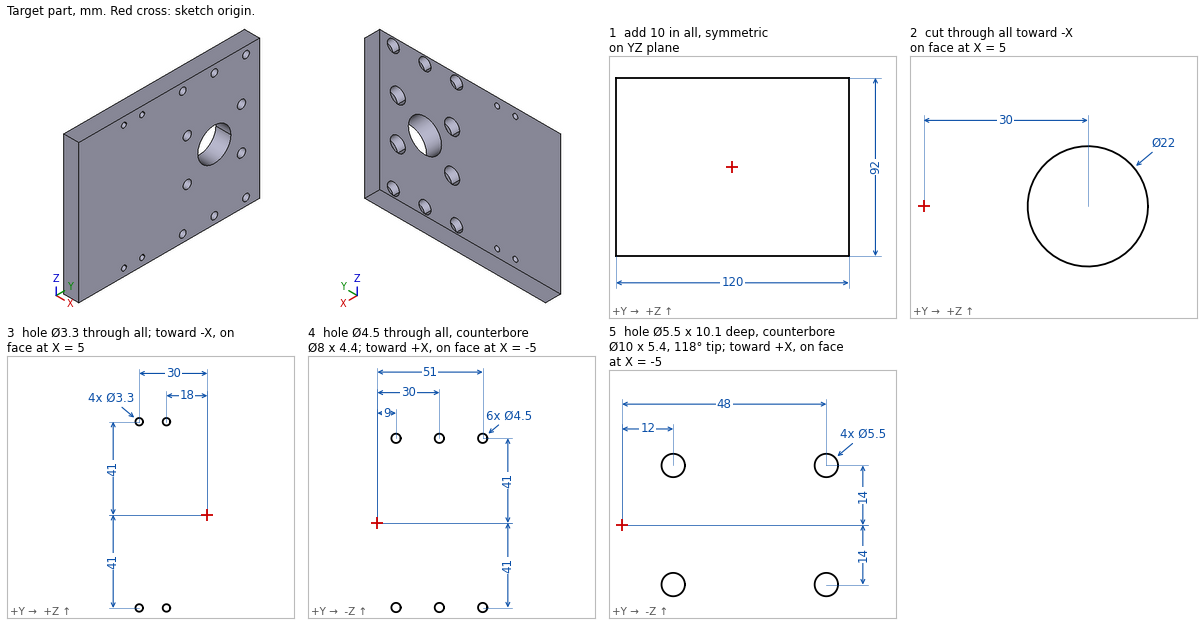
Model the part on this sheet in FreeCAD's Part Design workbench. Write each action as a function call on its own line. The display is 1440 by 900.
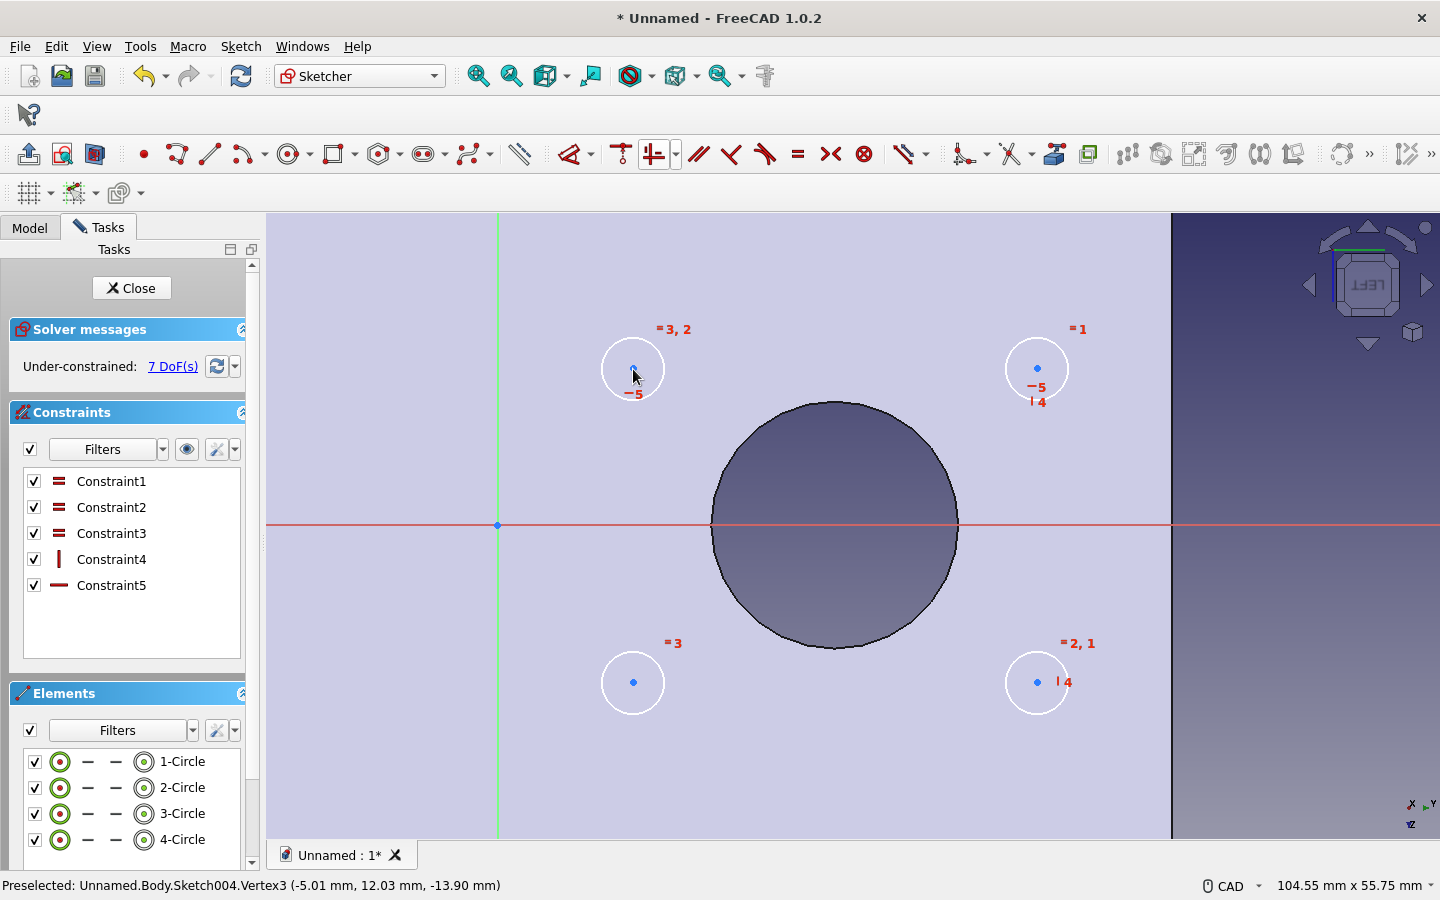
click(633, 369)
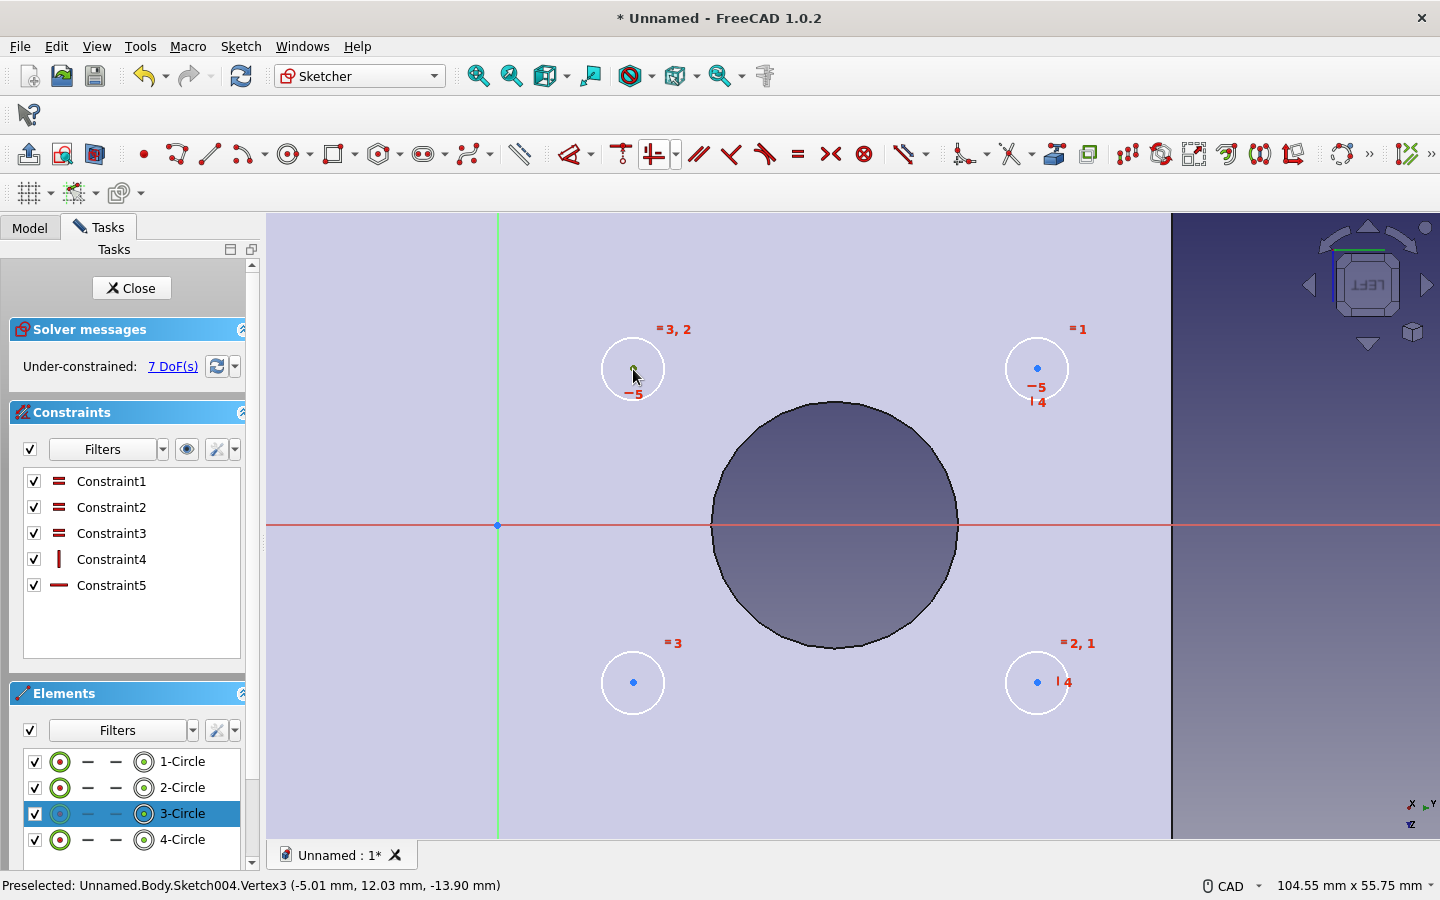
click(633, 683)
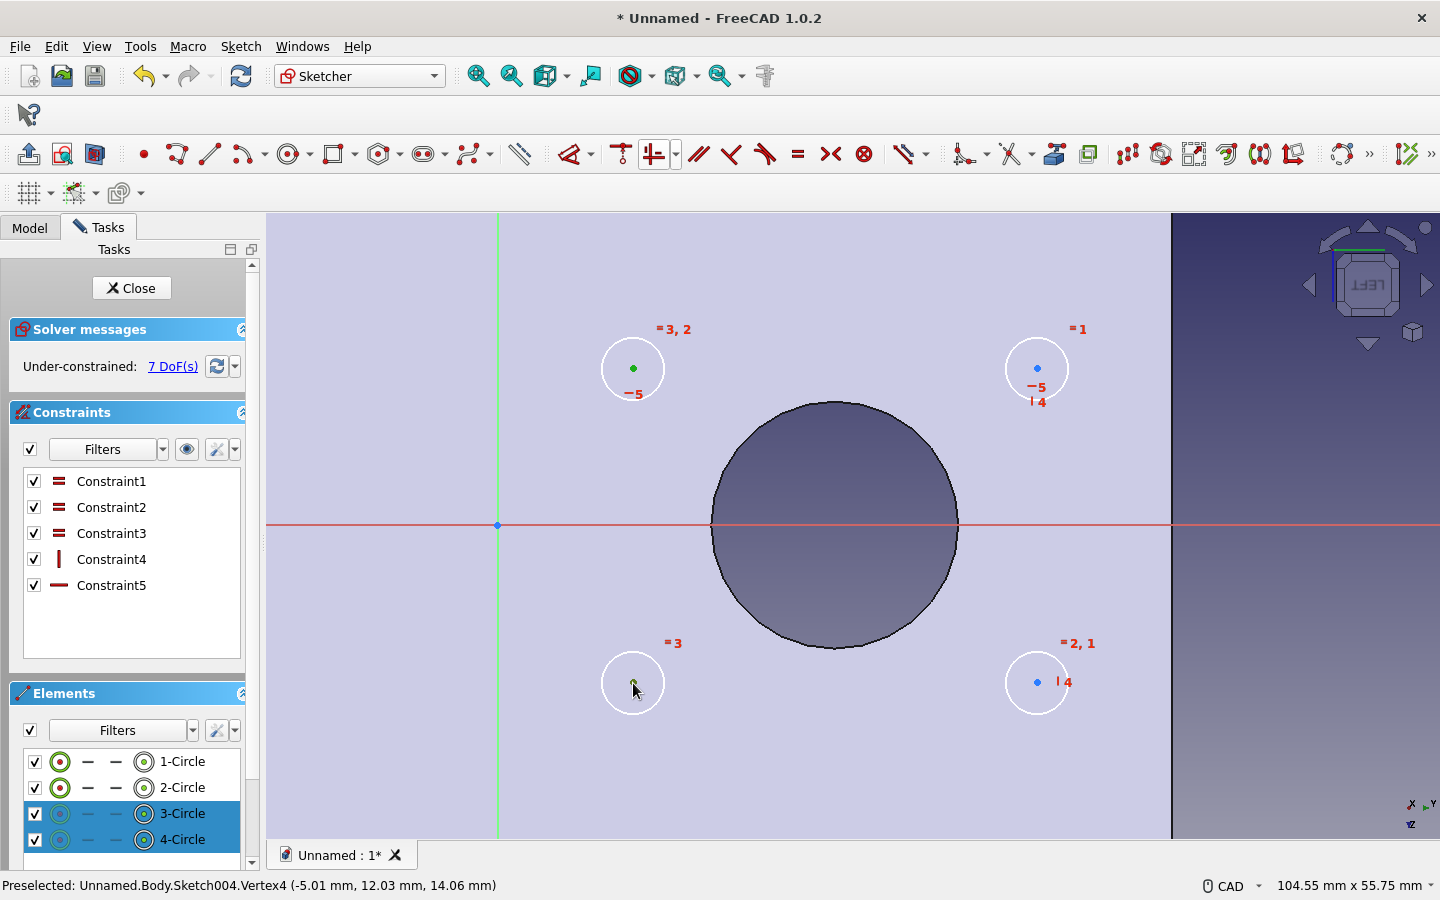
key(v)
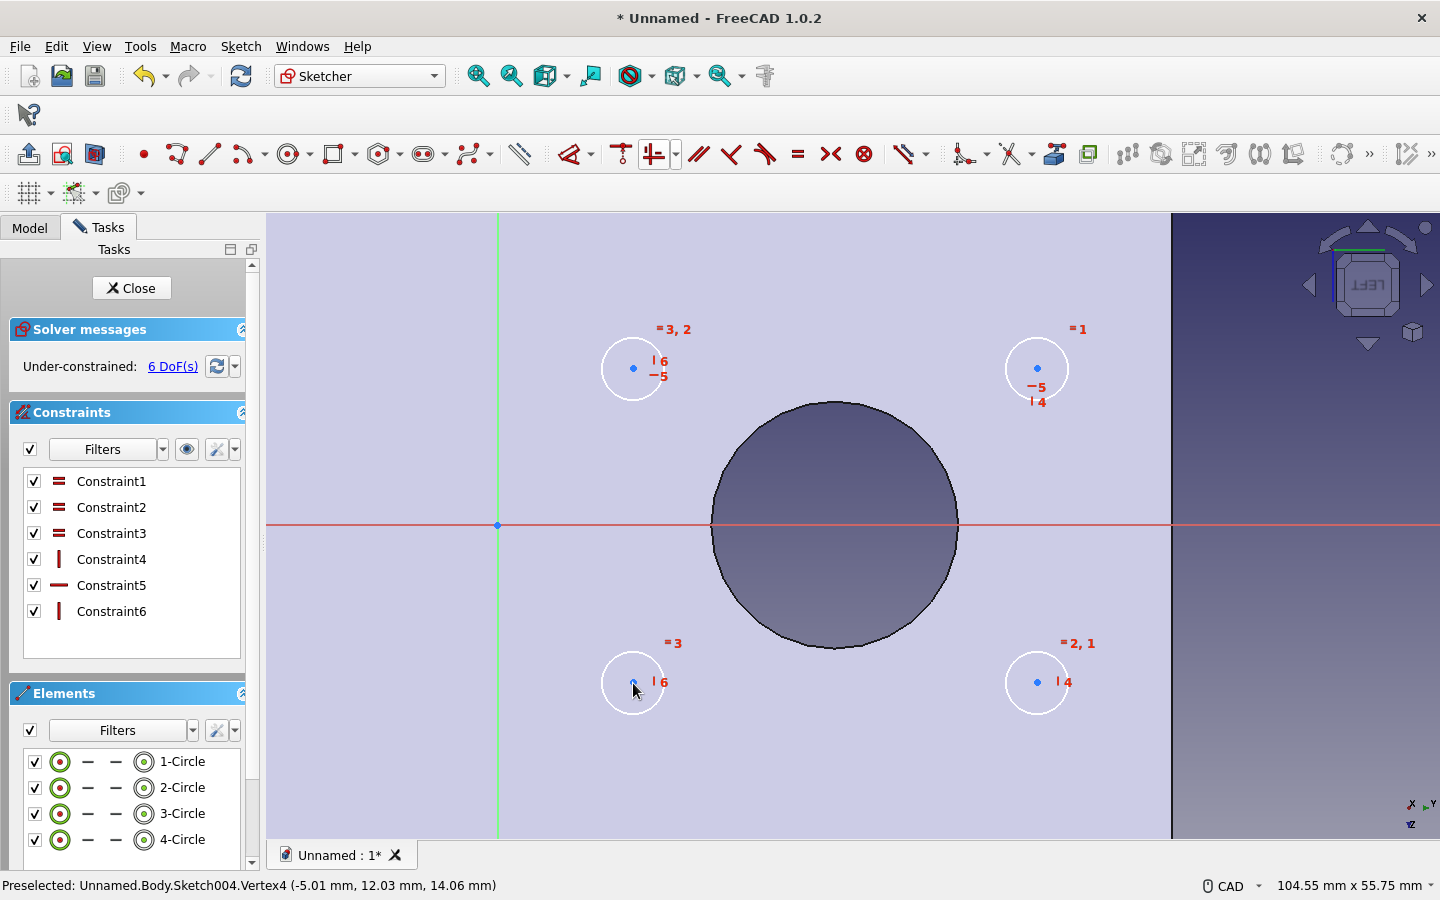
click(1037, 683)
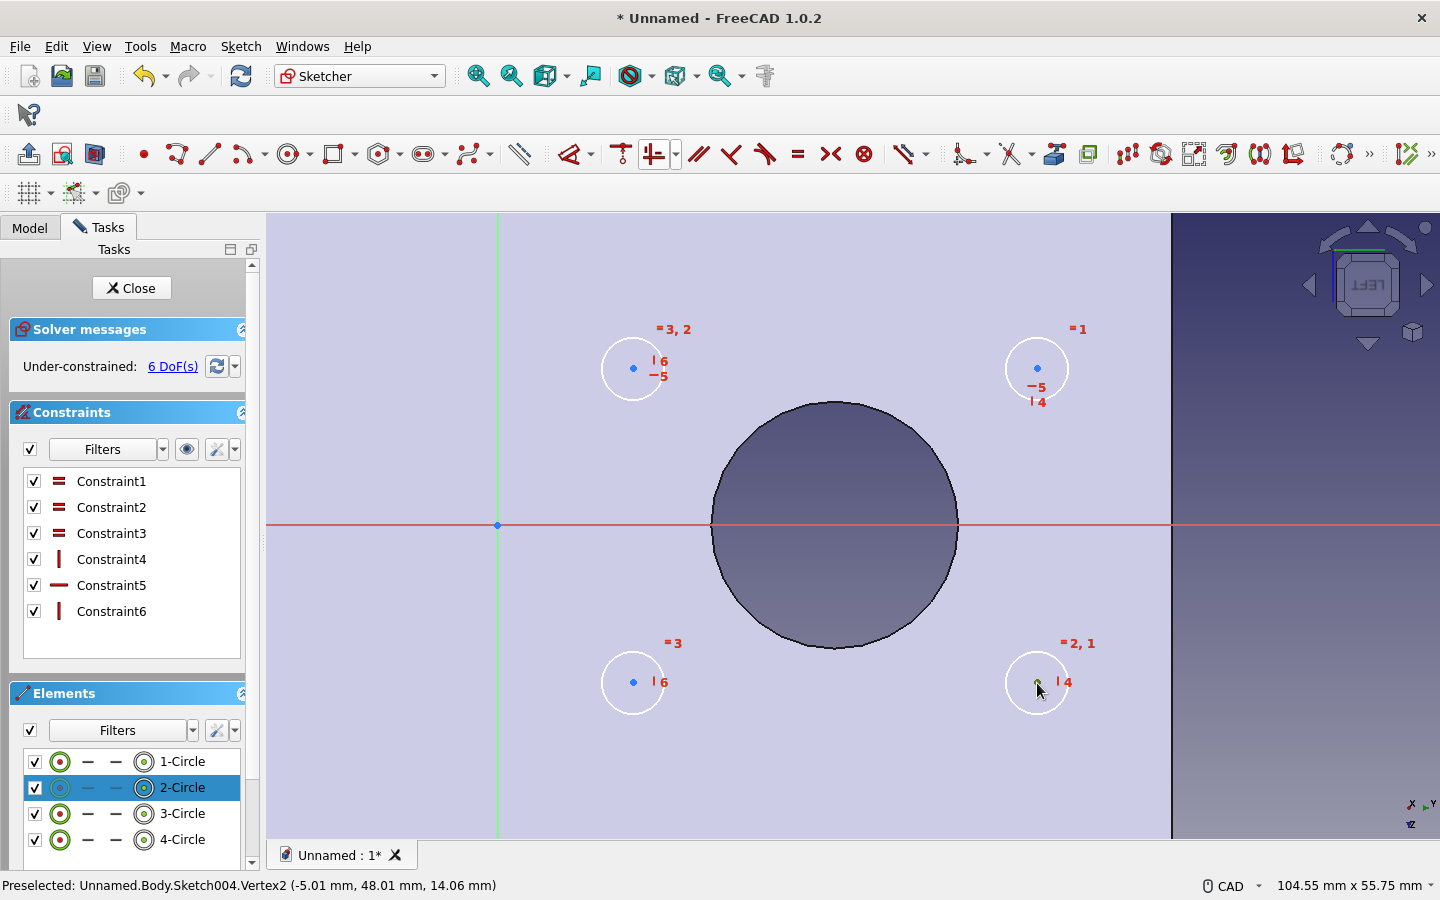
click(633, 683)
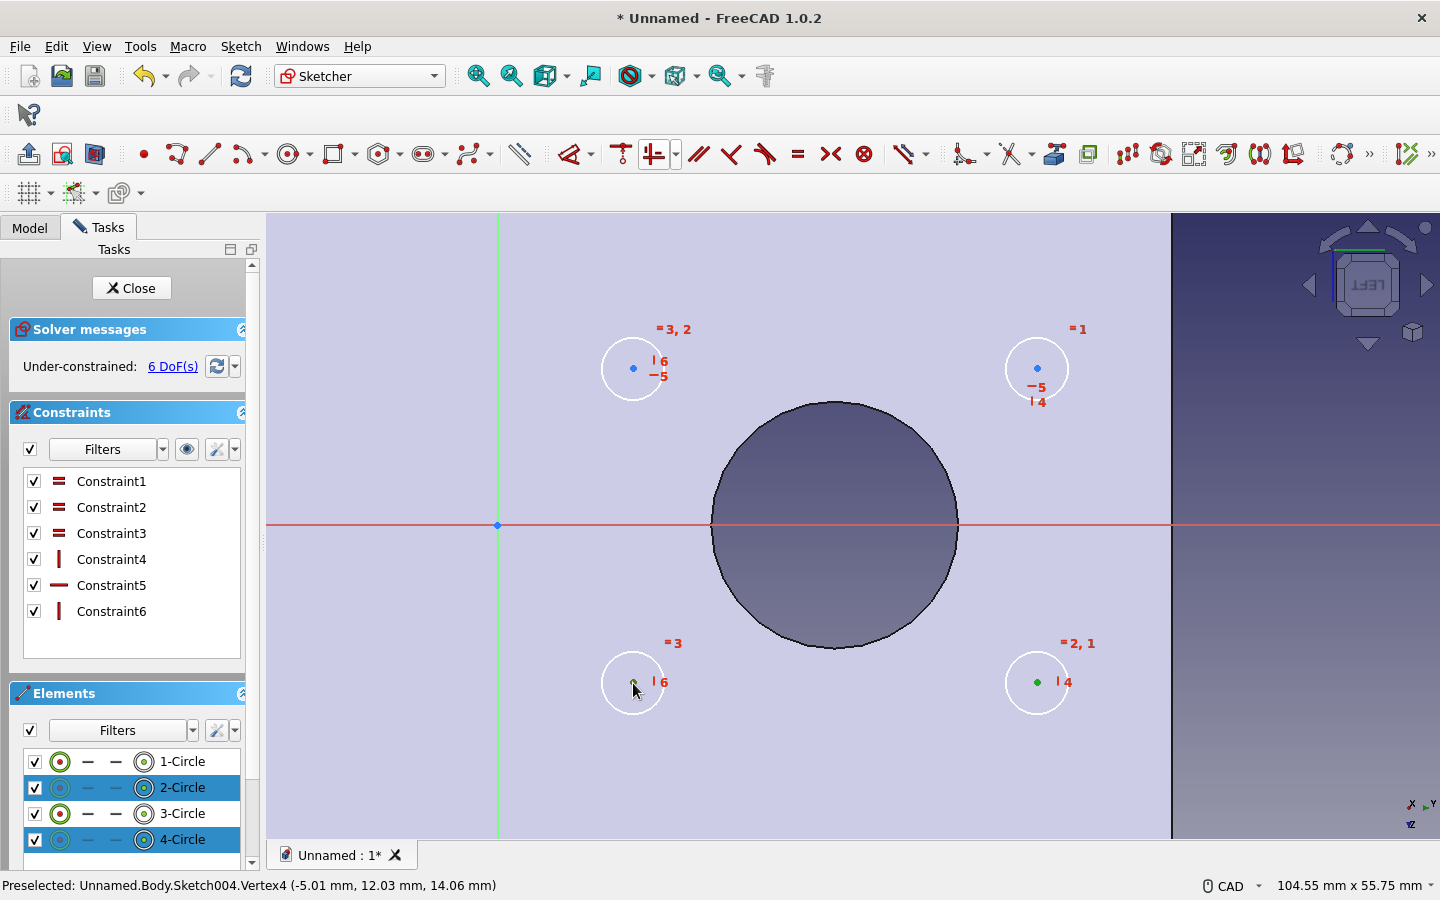
click(676, 154)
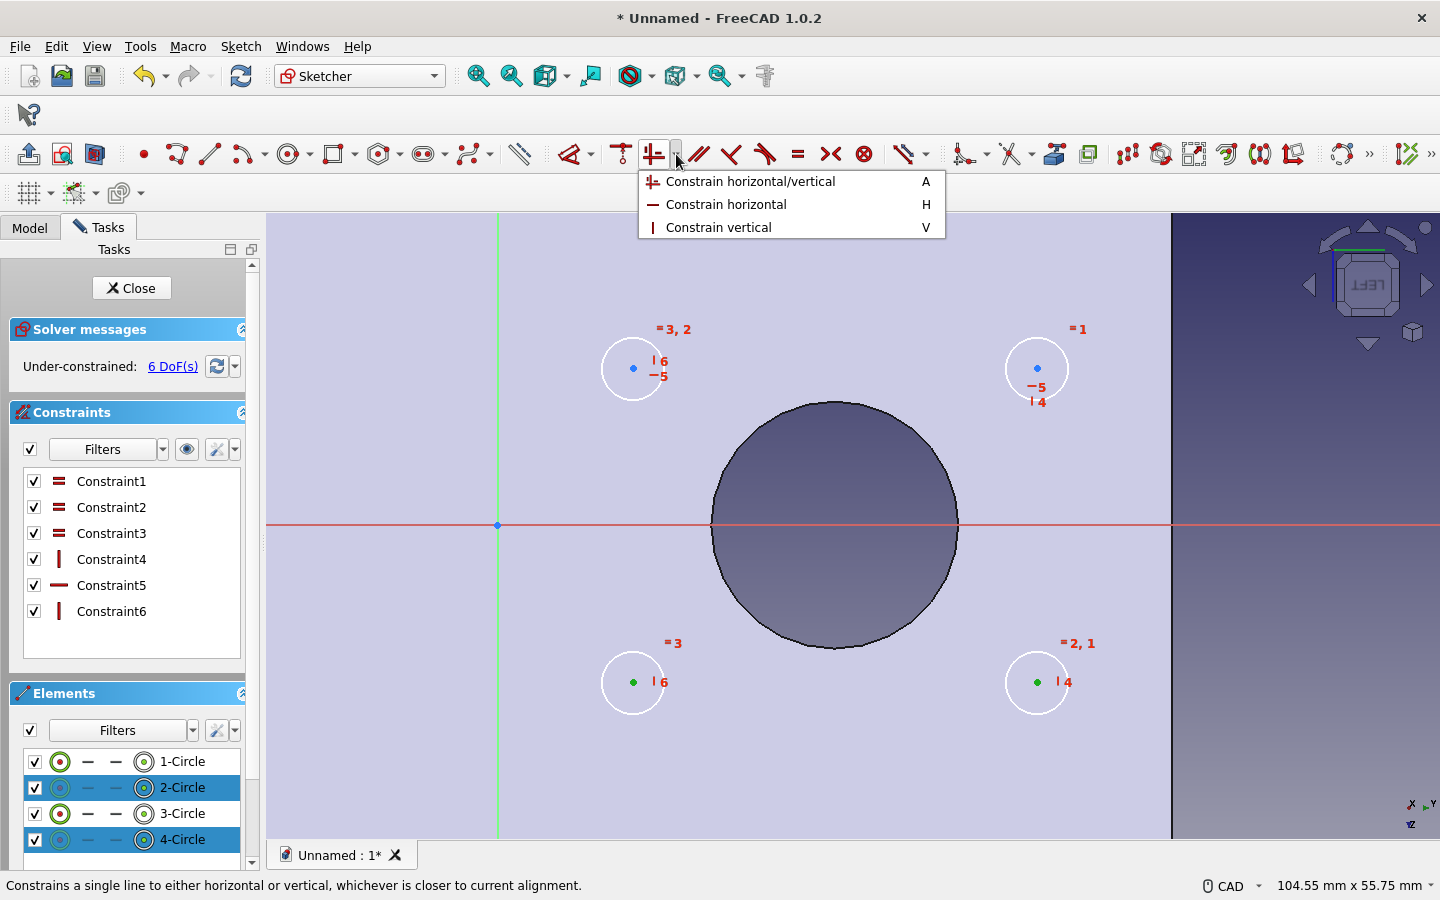
click(792, 204)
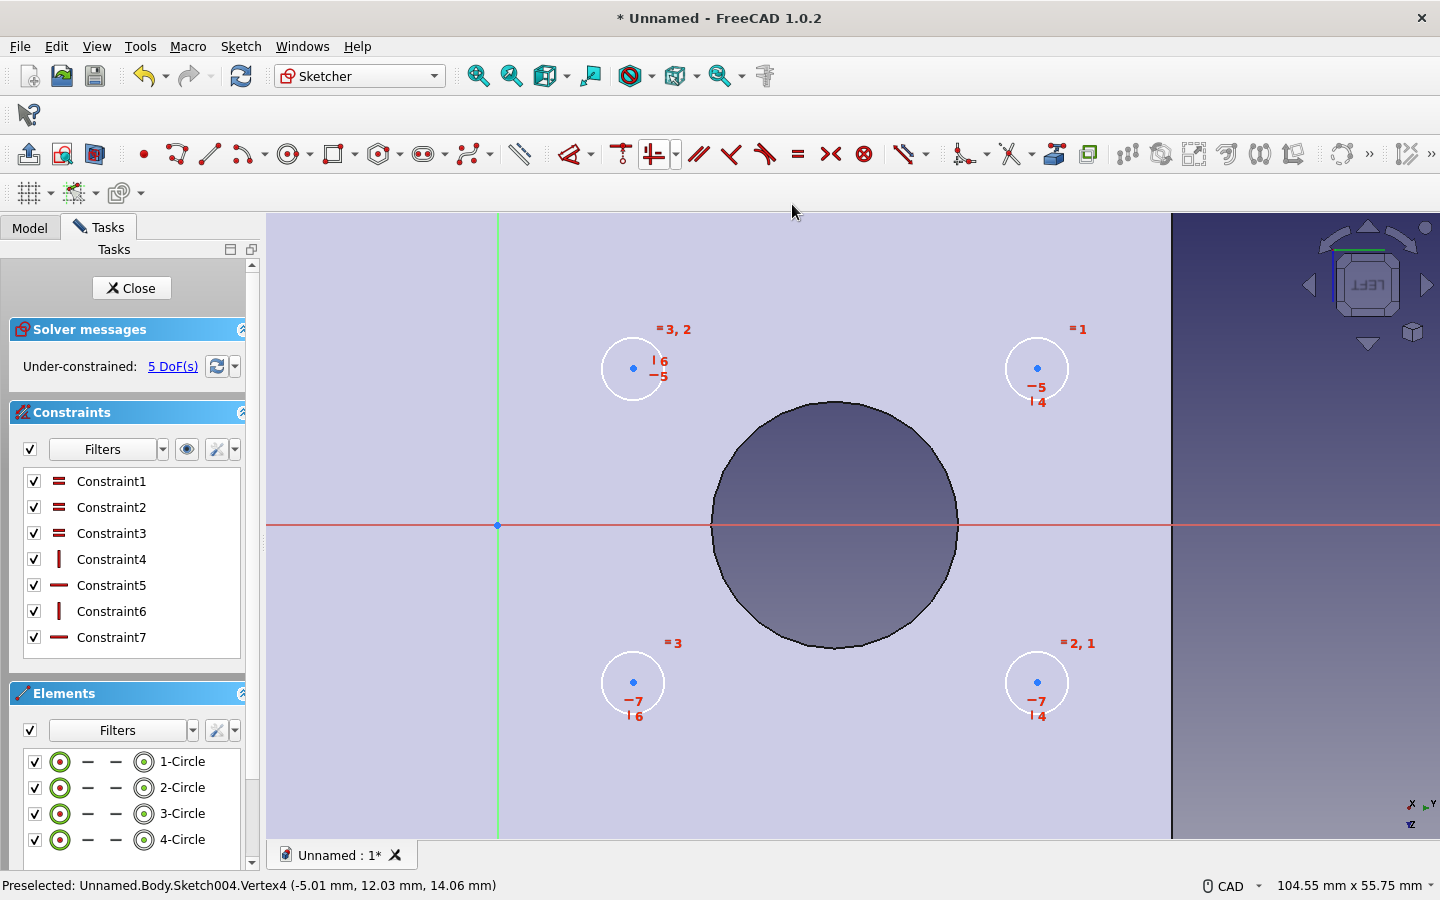
key(d)